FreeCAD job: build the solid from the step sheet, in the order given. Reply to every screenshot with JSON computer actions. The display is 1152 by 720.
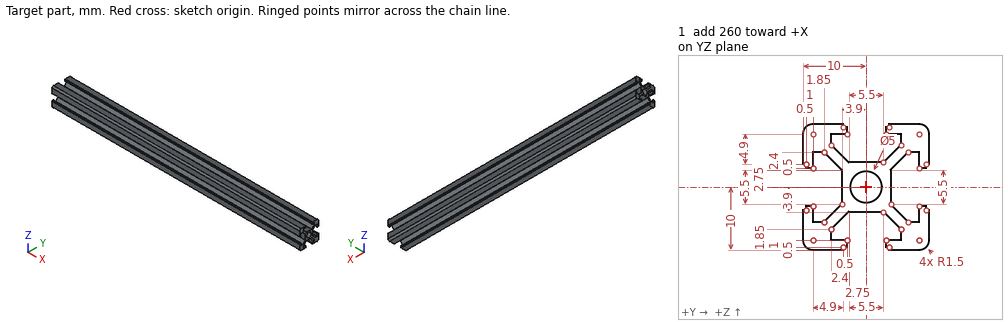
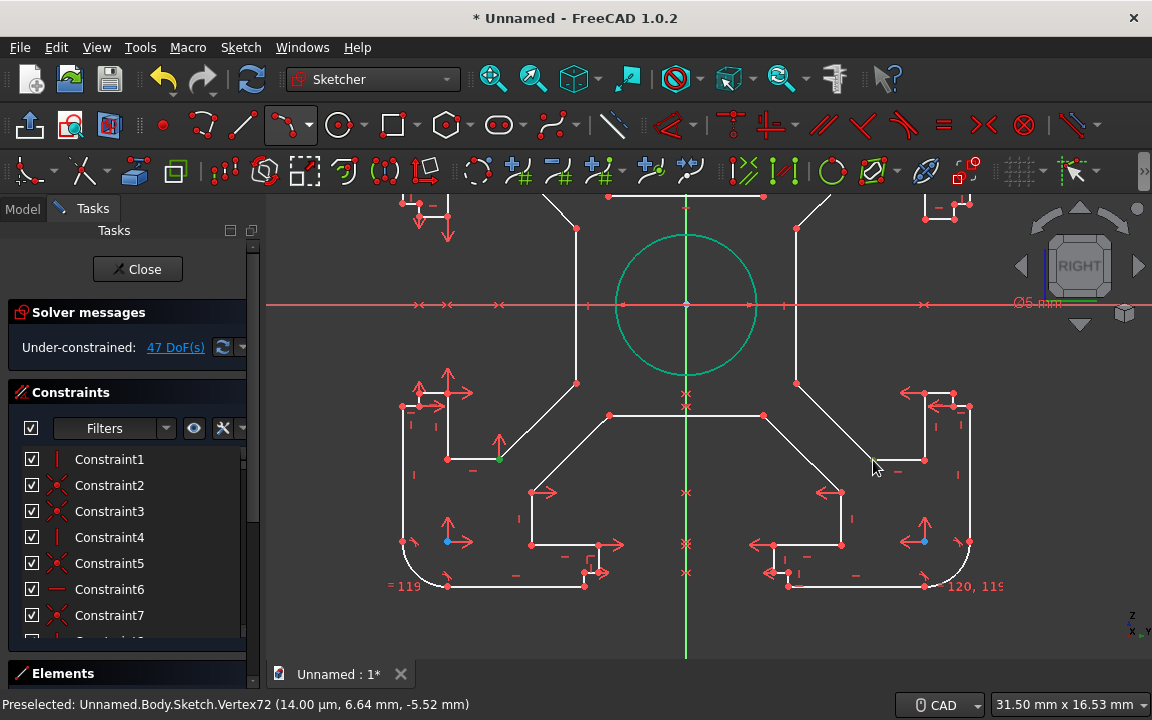
{"action": "left_click", "coordinate": [686, 602]}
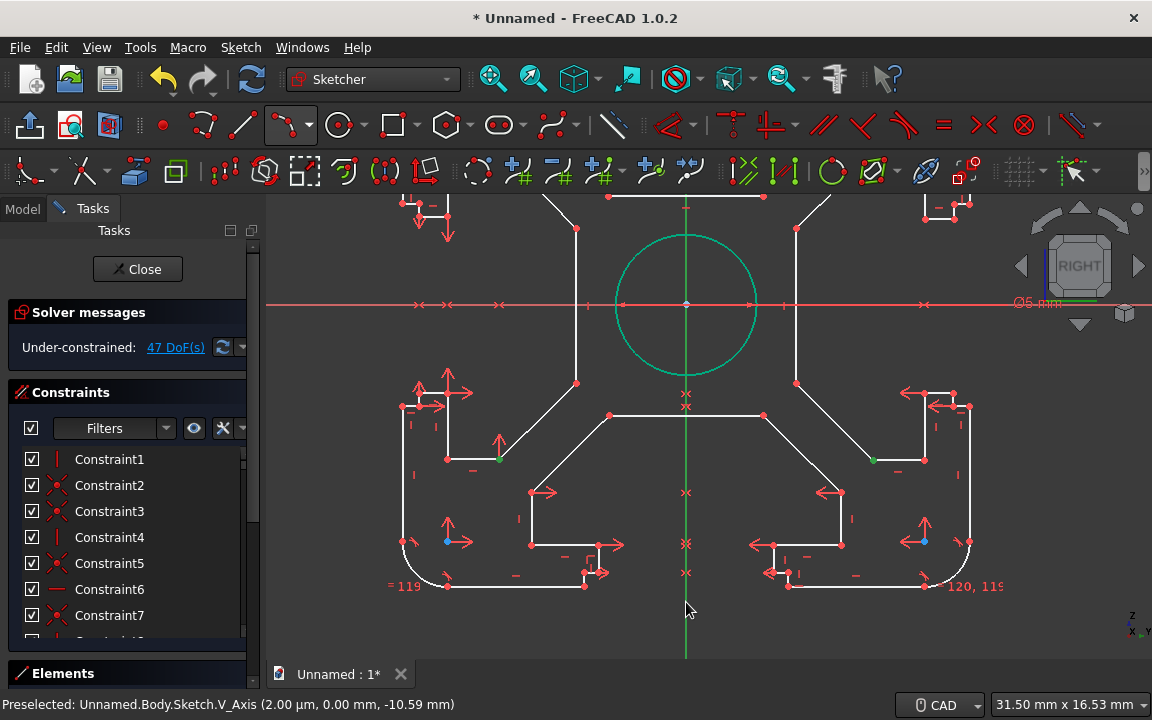
{"action": "key", "text": "s"}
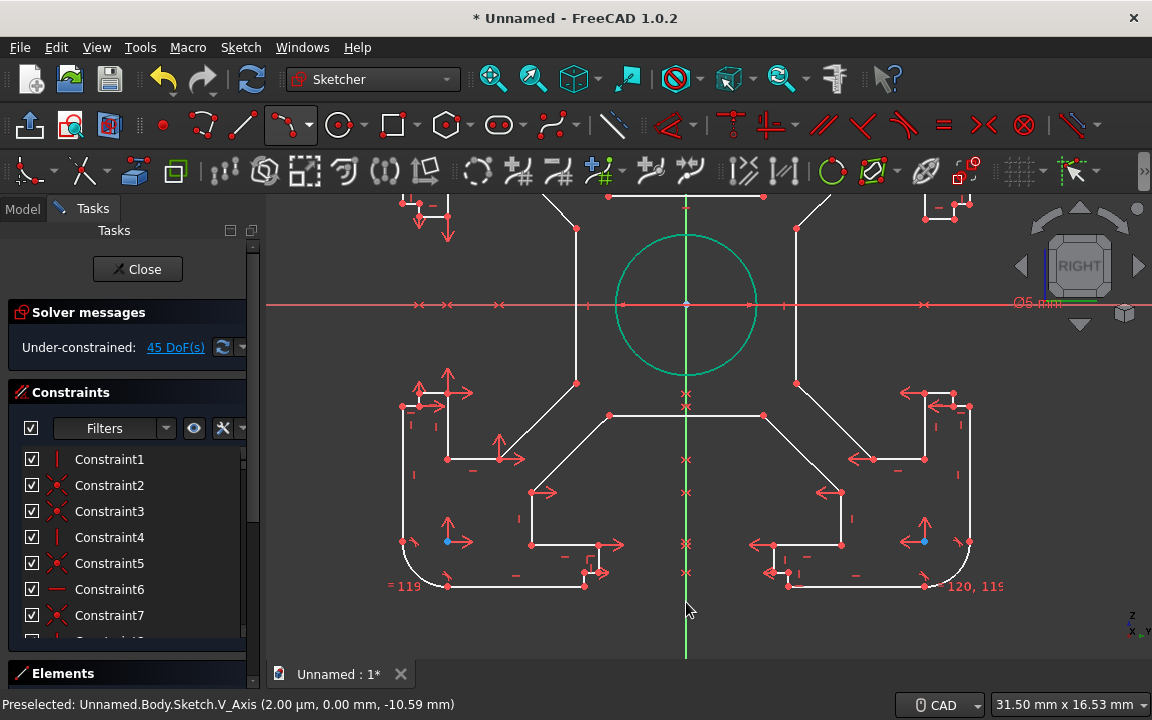
{"action": "left_click", "coordinate": [576, 383]}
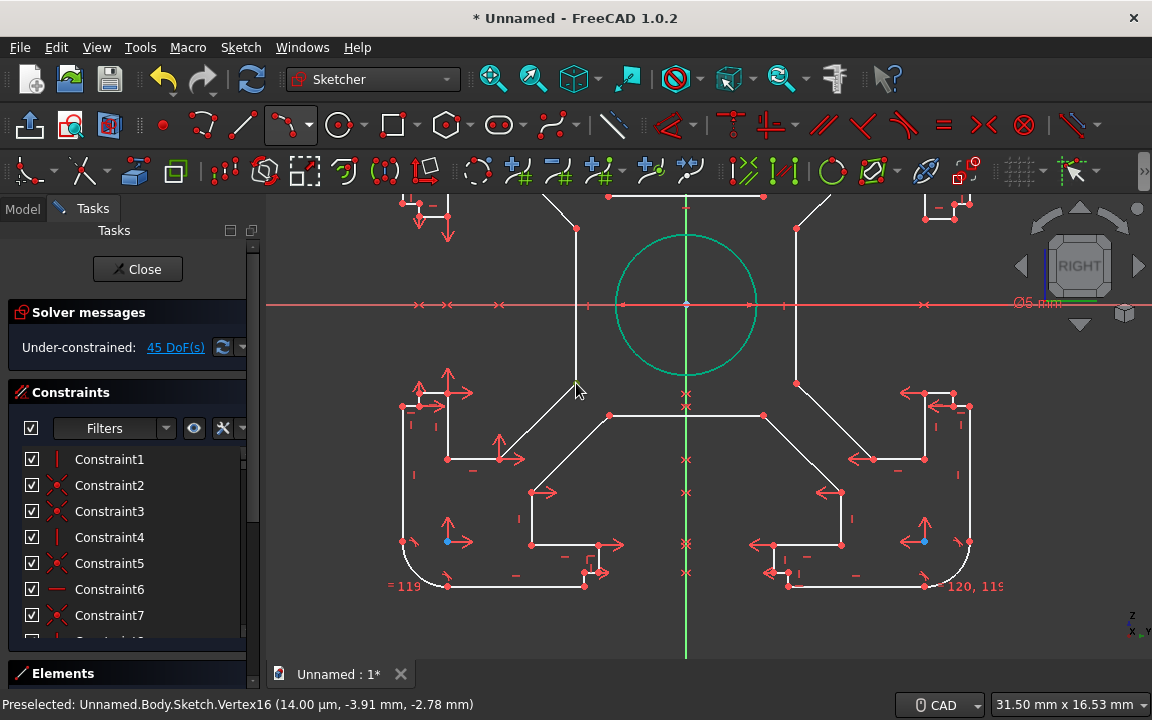
{"action": "left_click", "coordinate": [796, 383]}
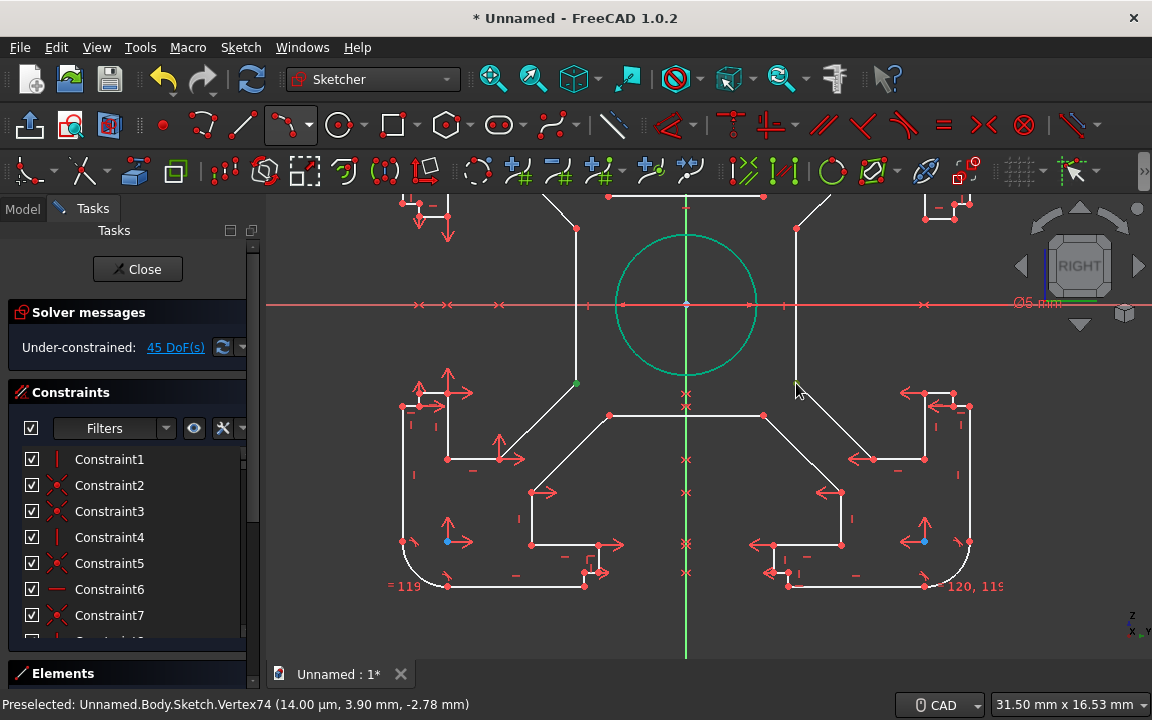
{"action": "left_click", "coordinate": [686, 602]}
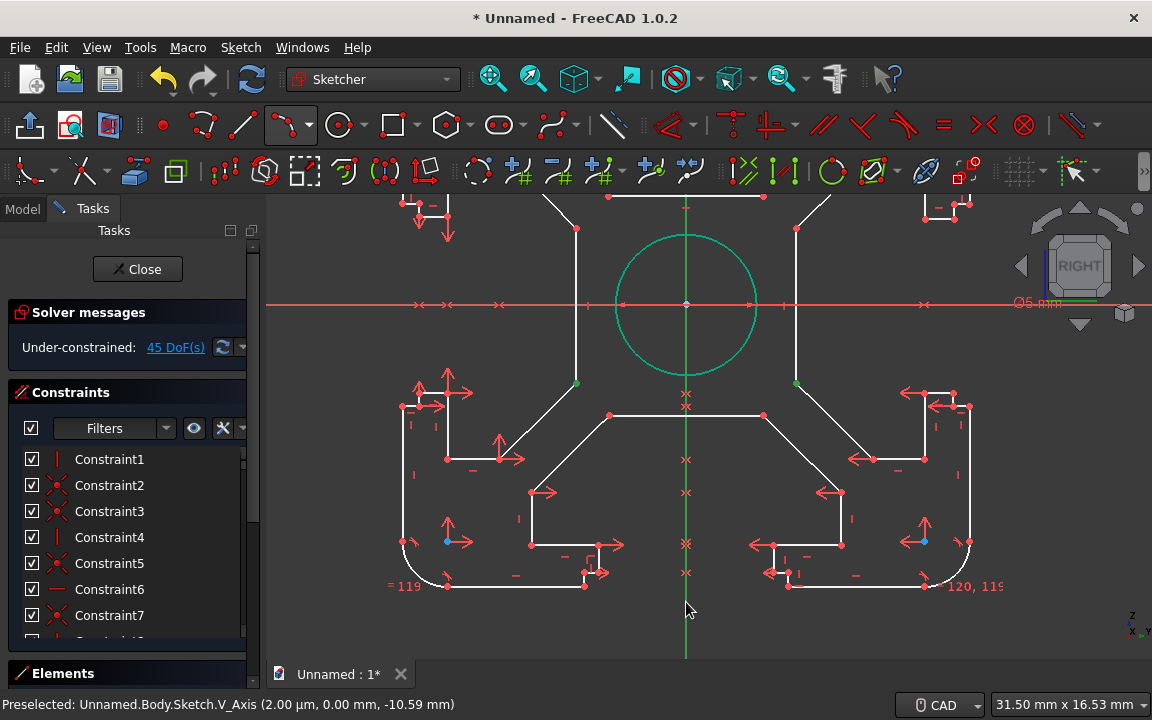
{"action": "left_click", "coordinate": [984, 126]}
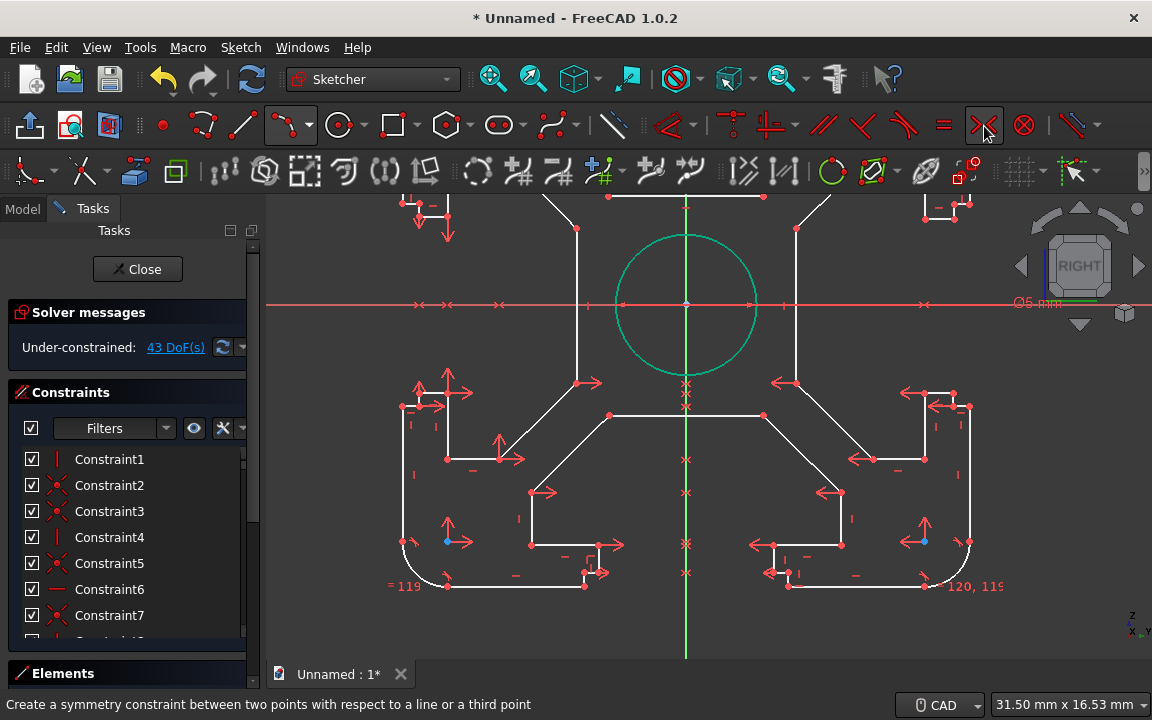
{"action": "scroll", "coordinate": [585, 574], "scroll_direction": "down", "scroll_amount": 3}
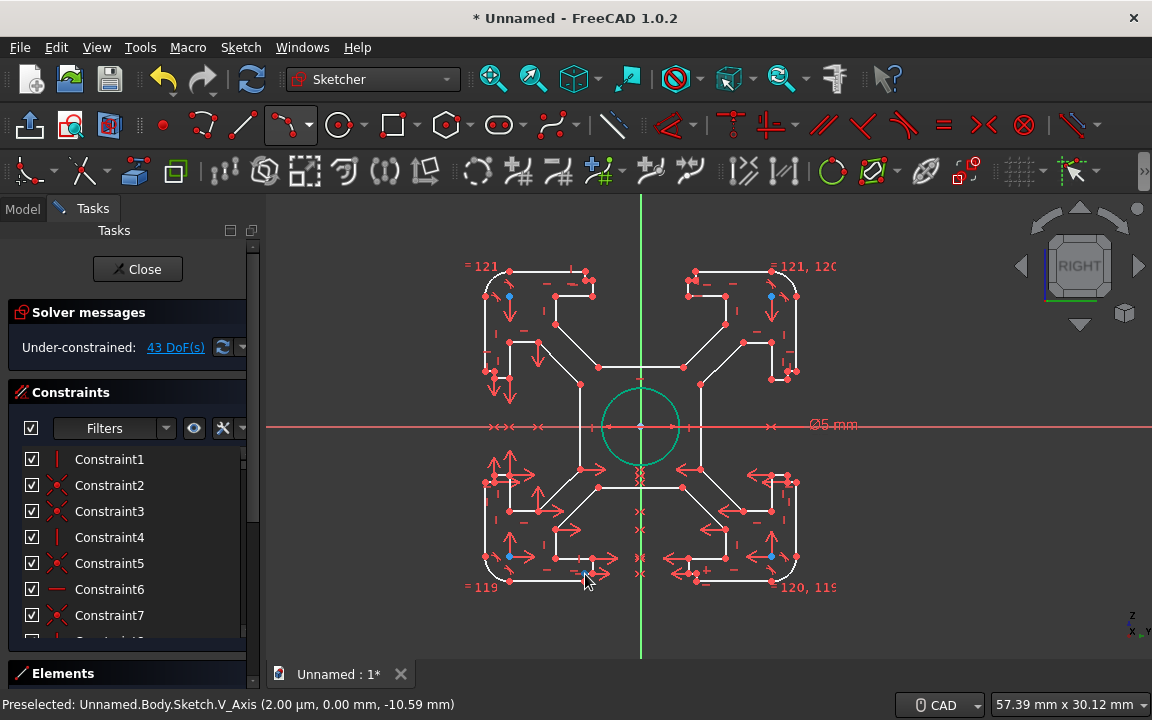
{"action": "left_click", "coordinate": [538, 342]}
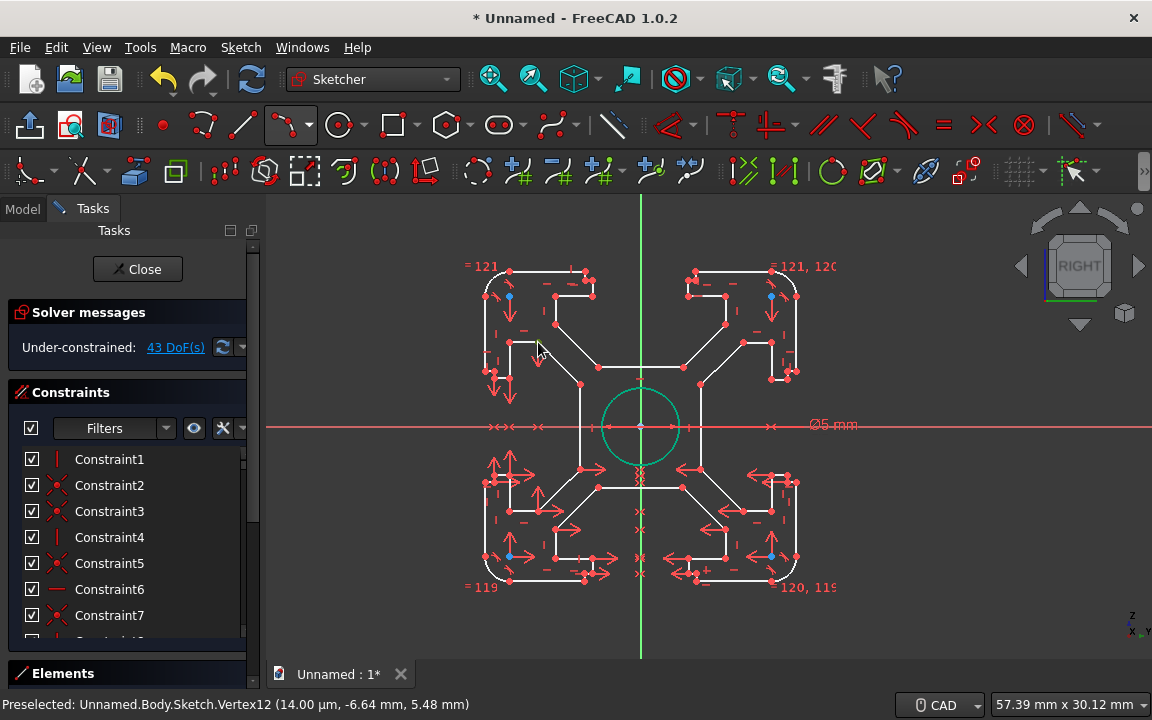
{"action": "left_click", "coordinate": [744, 343]}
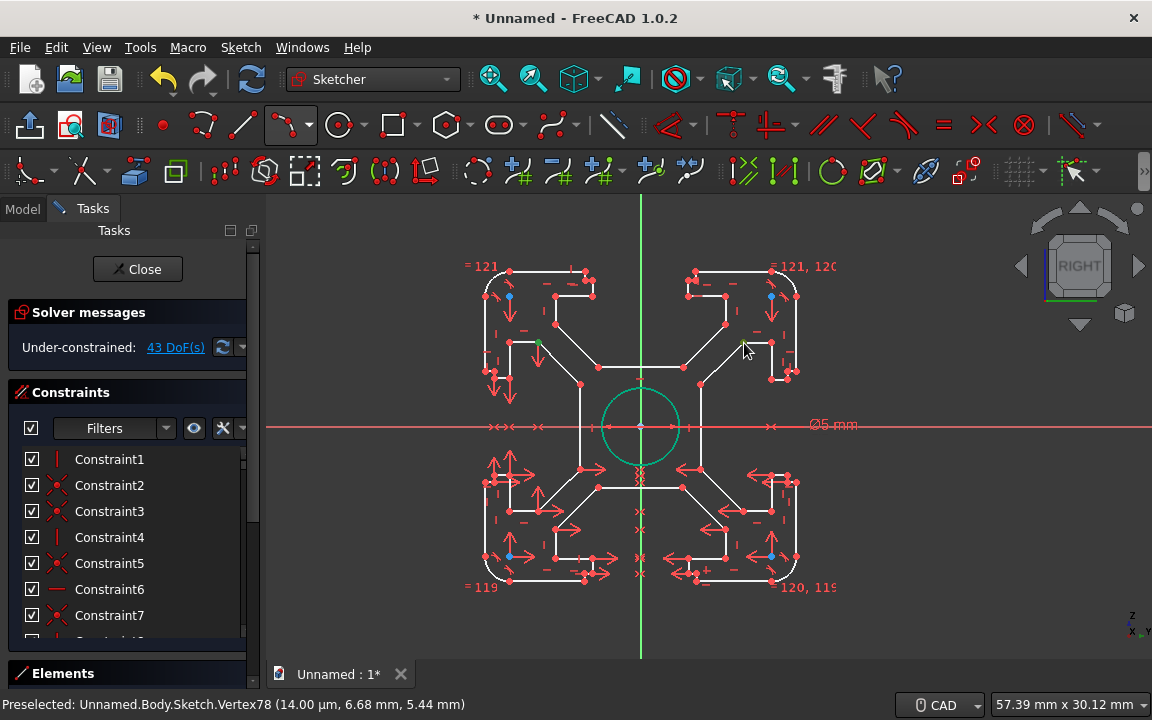
{"action": "left_click", "coordinate": [641, 602]}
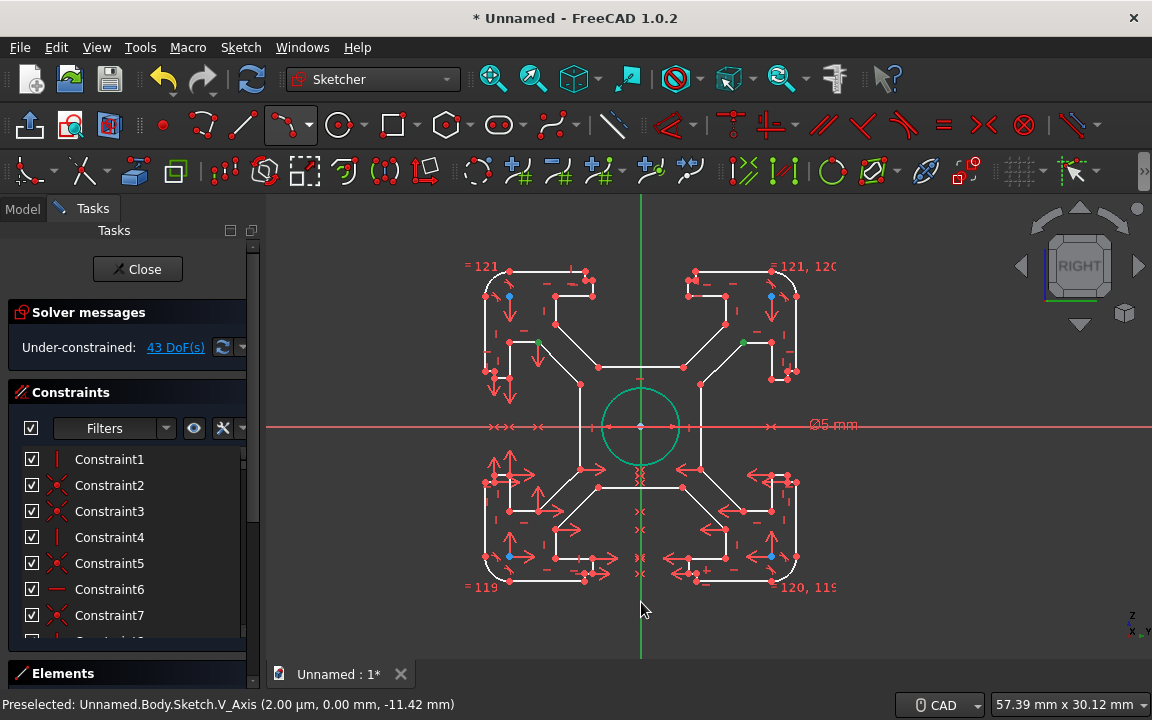
{"action": "key", "text": "s"}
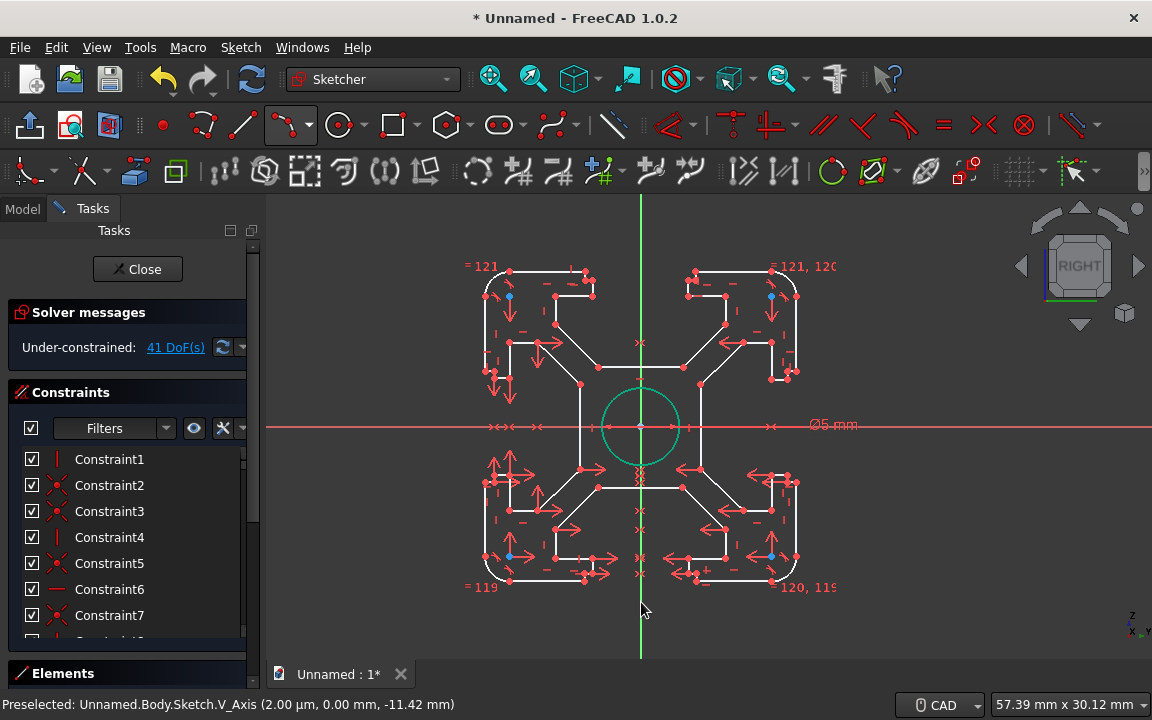
{"action": "left_click", "coordinate": [510, 378]}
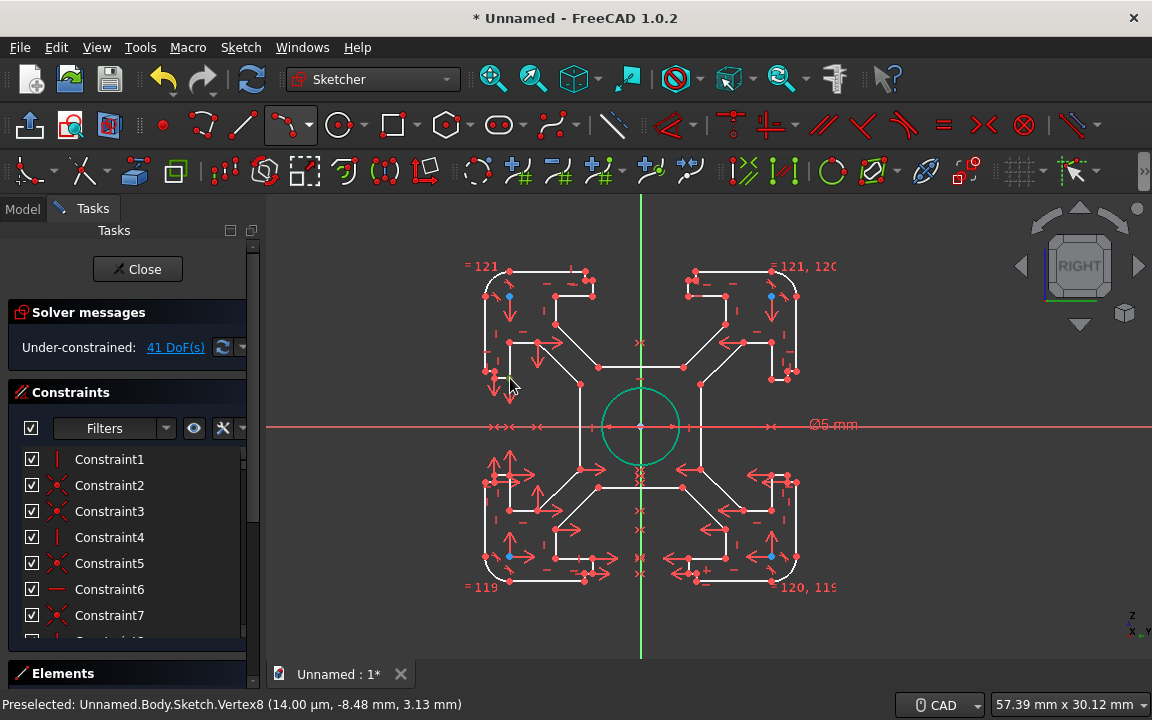
{"action": "left_click", "coordinate": [772, 380]}